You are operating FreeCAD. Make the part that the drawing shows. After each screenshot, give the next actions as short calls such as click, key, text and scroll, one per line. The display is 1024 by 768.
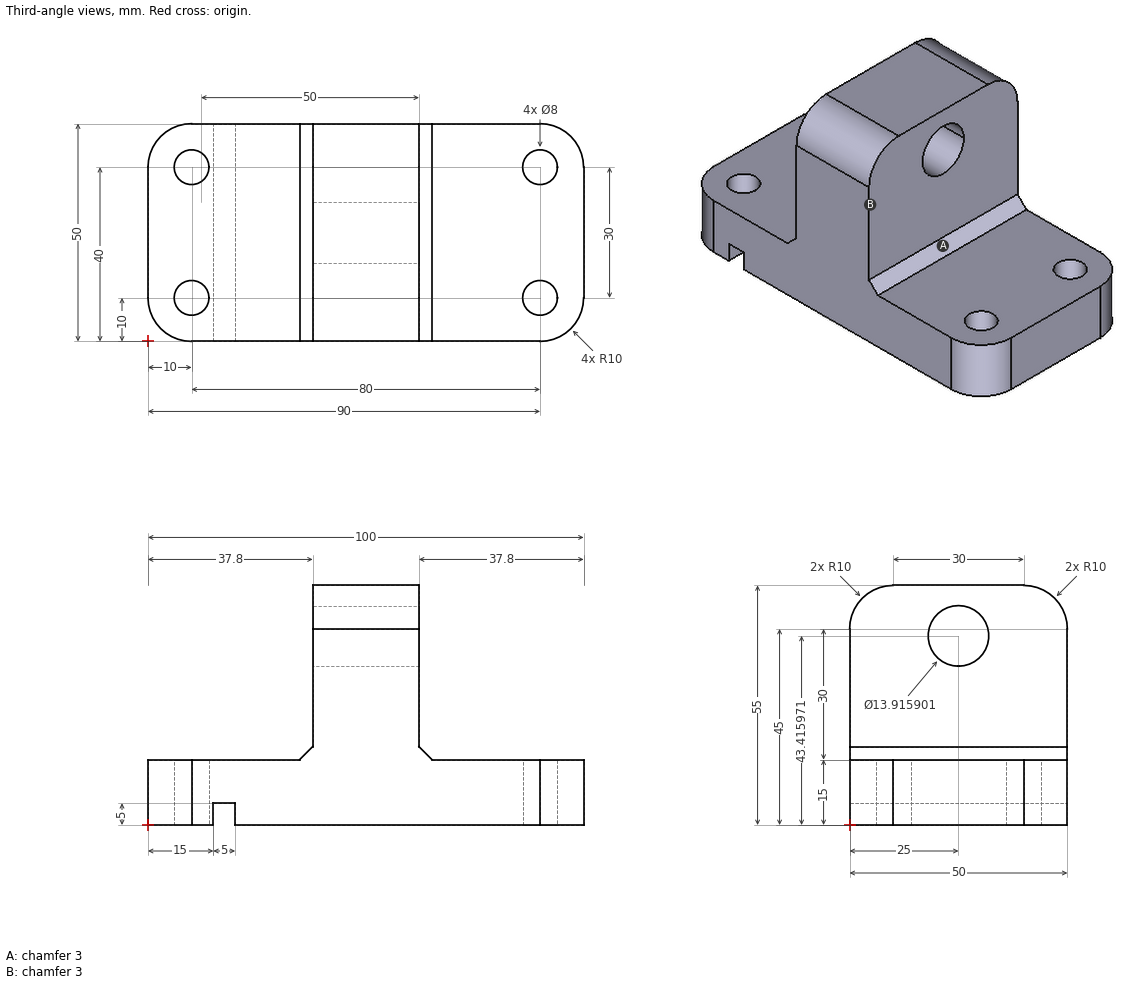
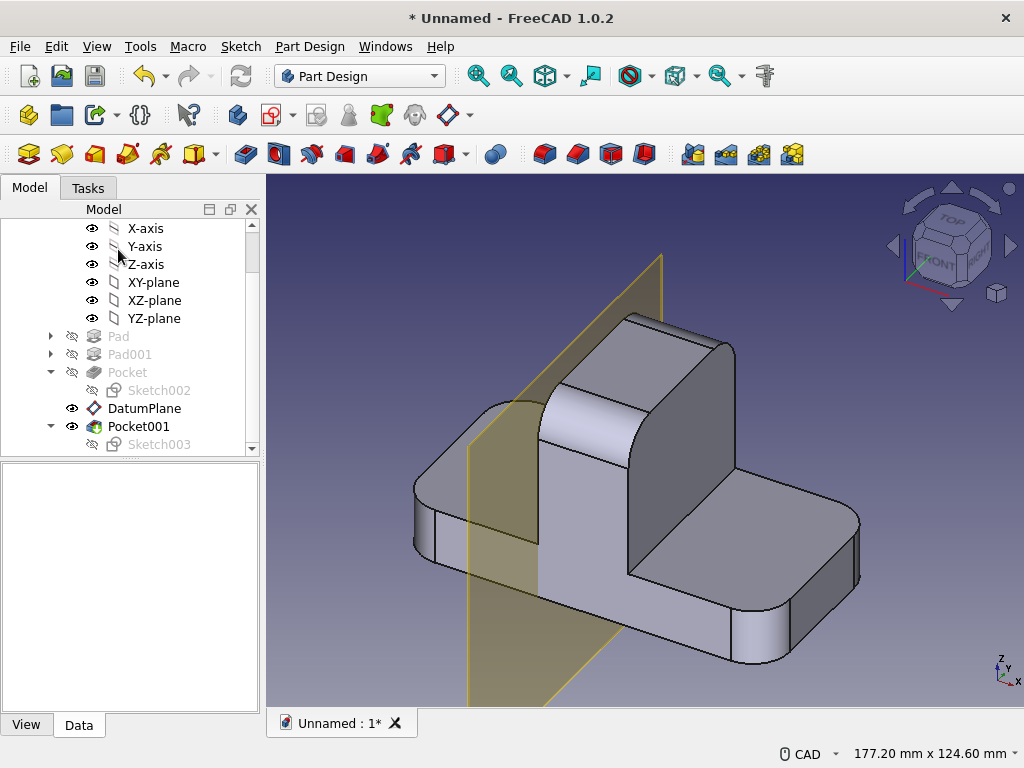
click(117, 408)
key(space)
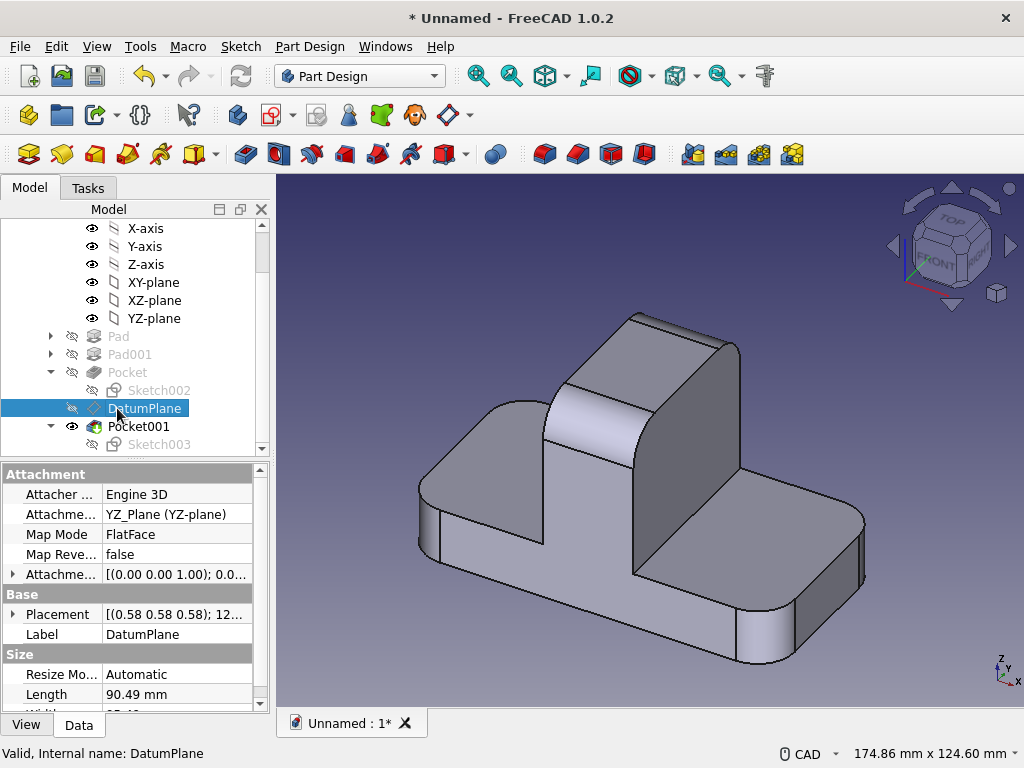
click(316, 667)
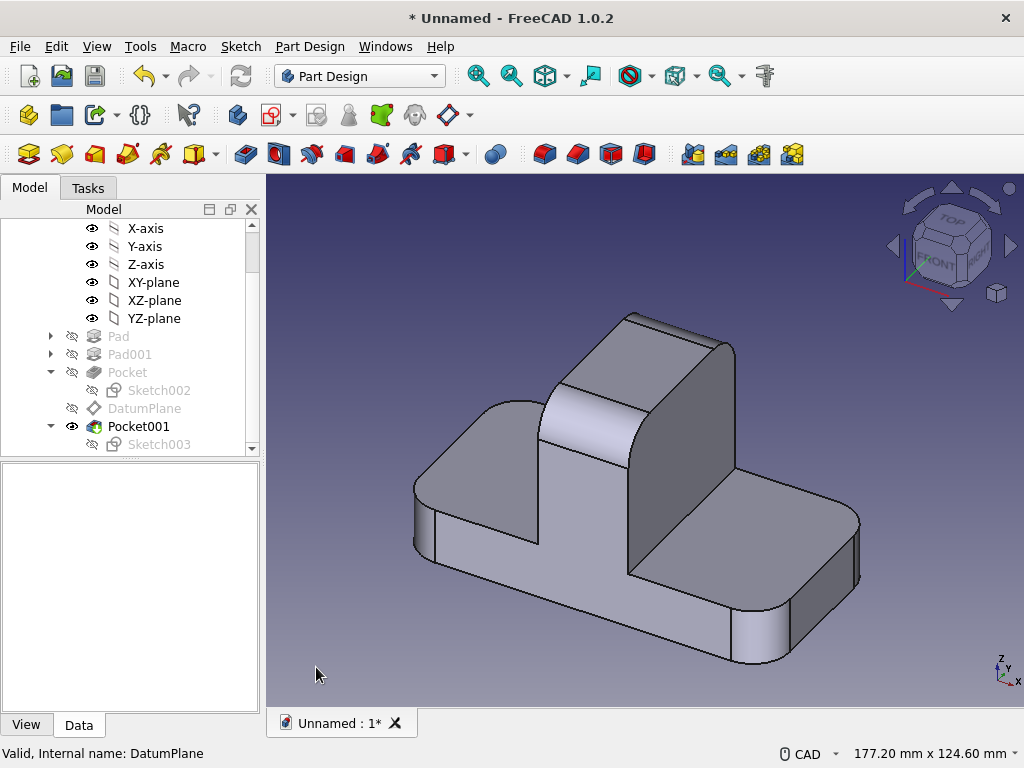
click(270, 116)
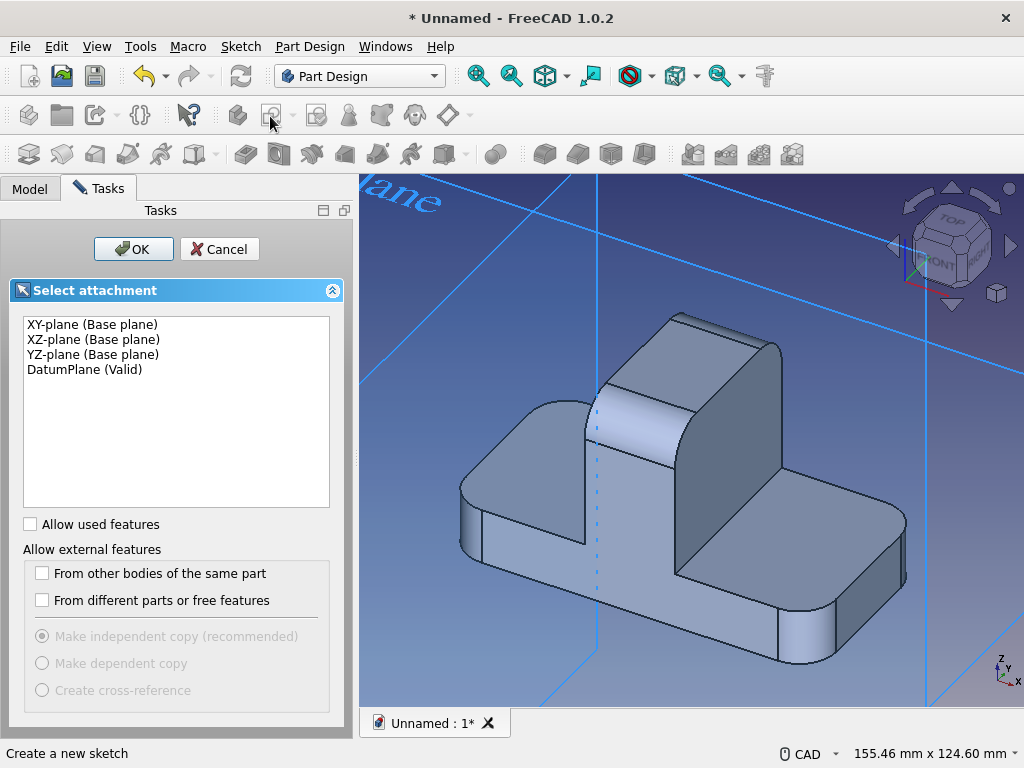
click(84, 340)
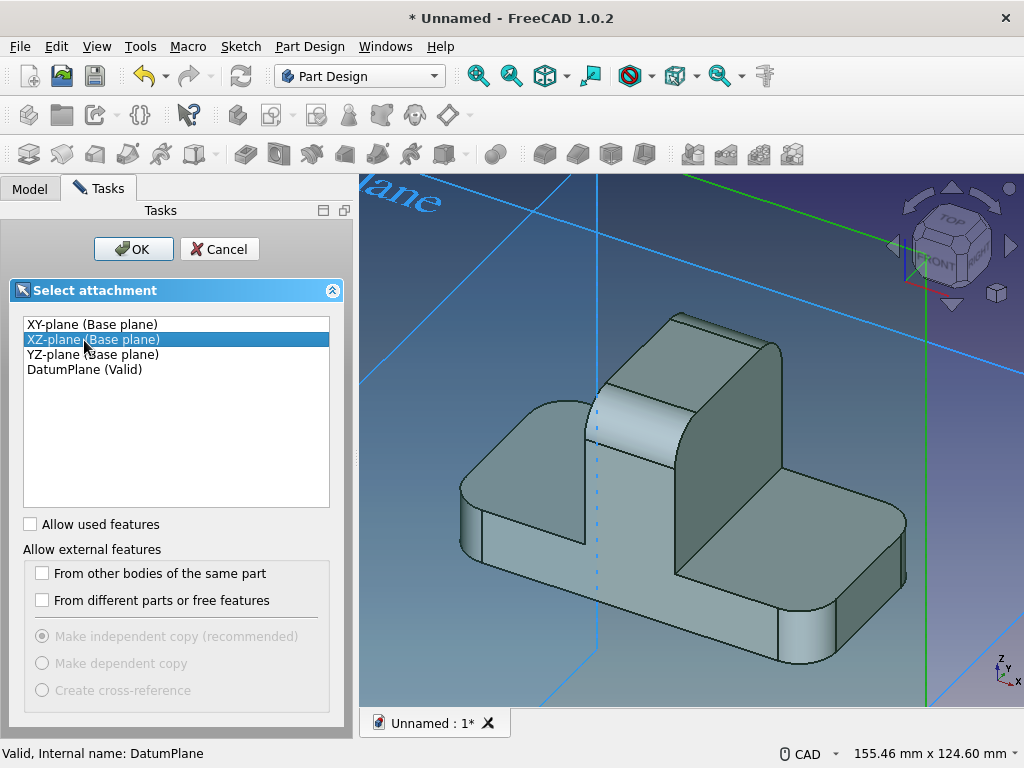
click(134, 249)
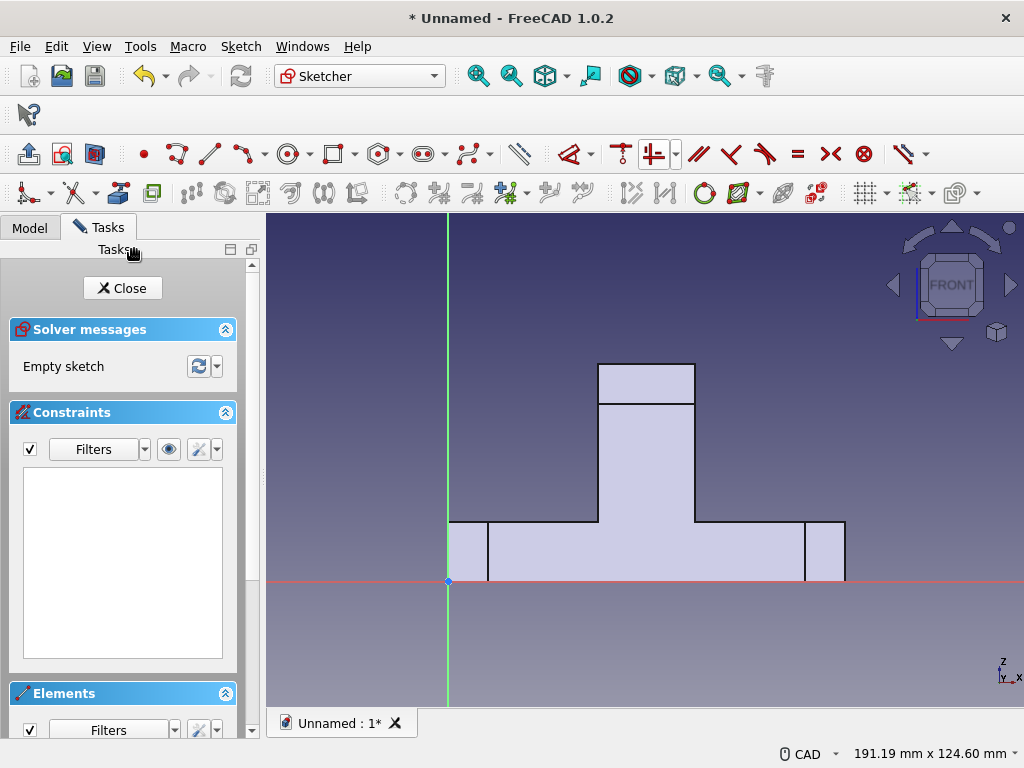
scroll(514, 579, up, 14)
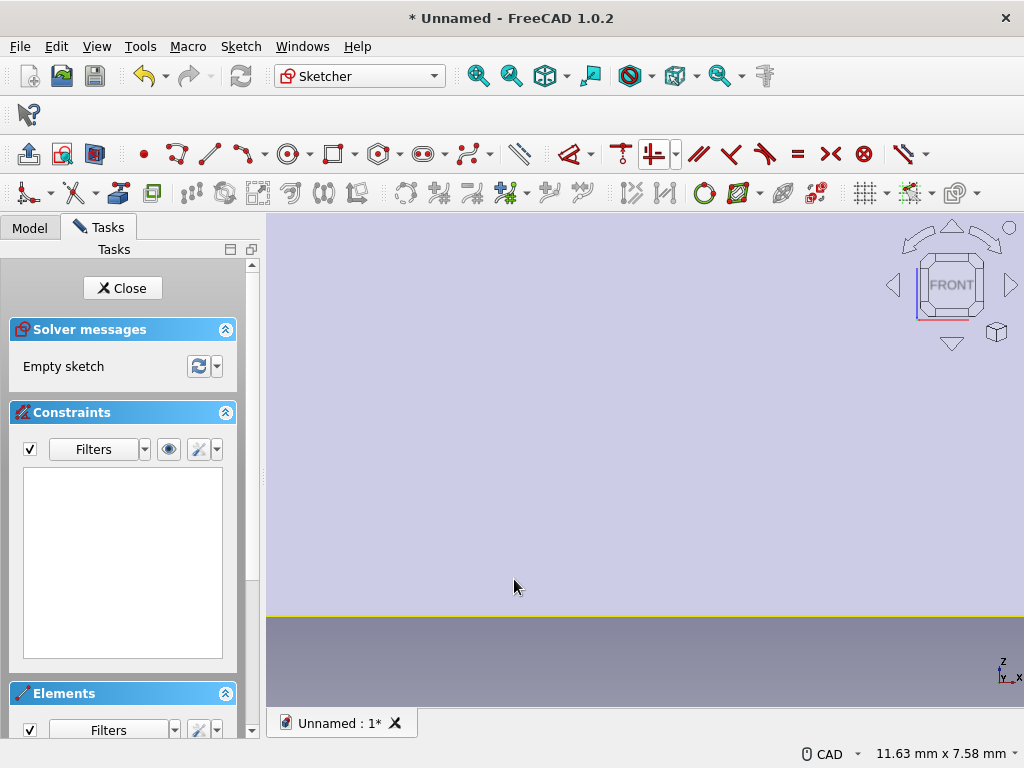
click(332, 154)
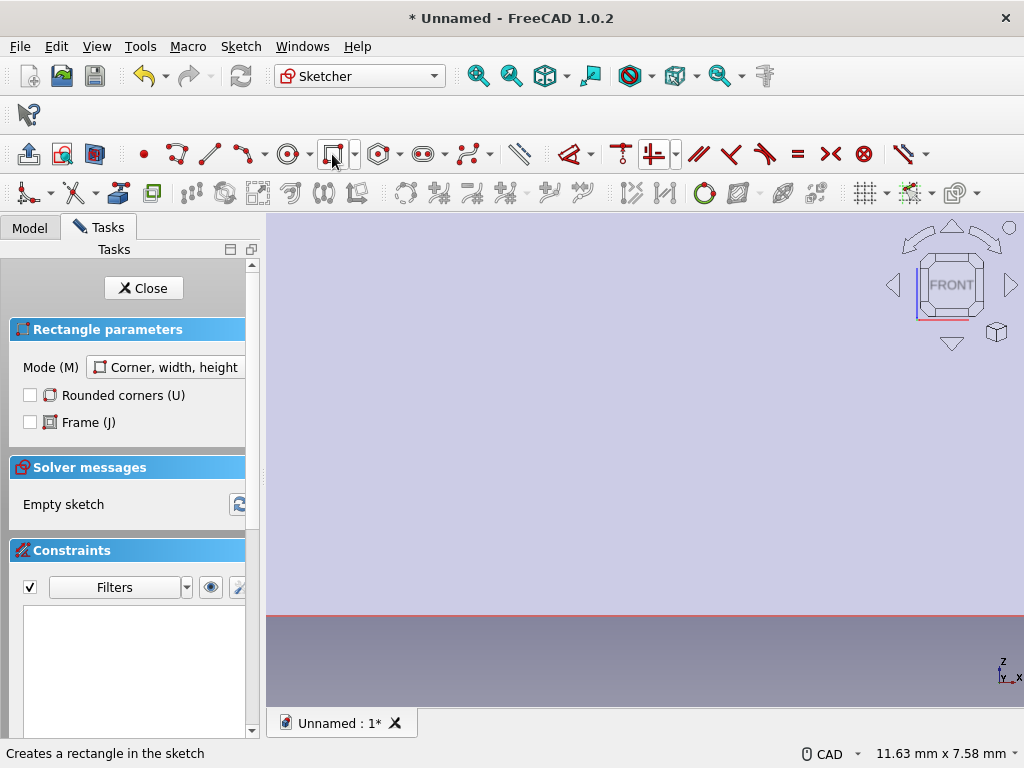
click(409, 290)
click(735, 616)
key(Escape)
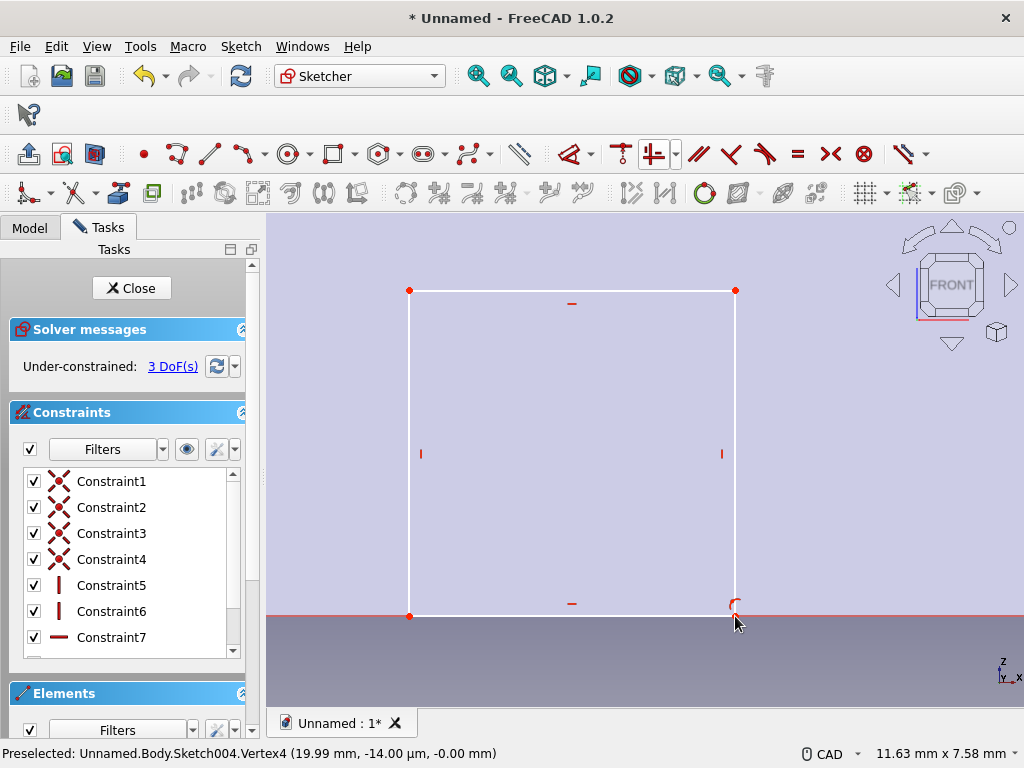
click(568, 154)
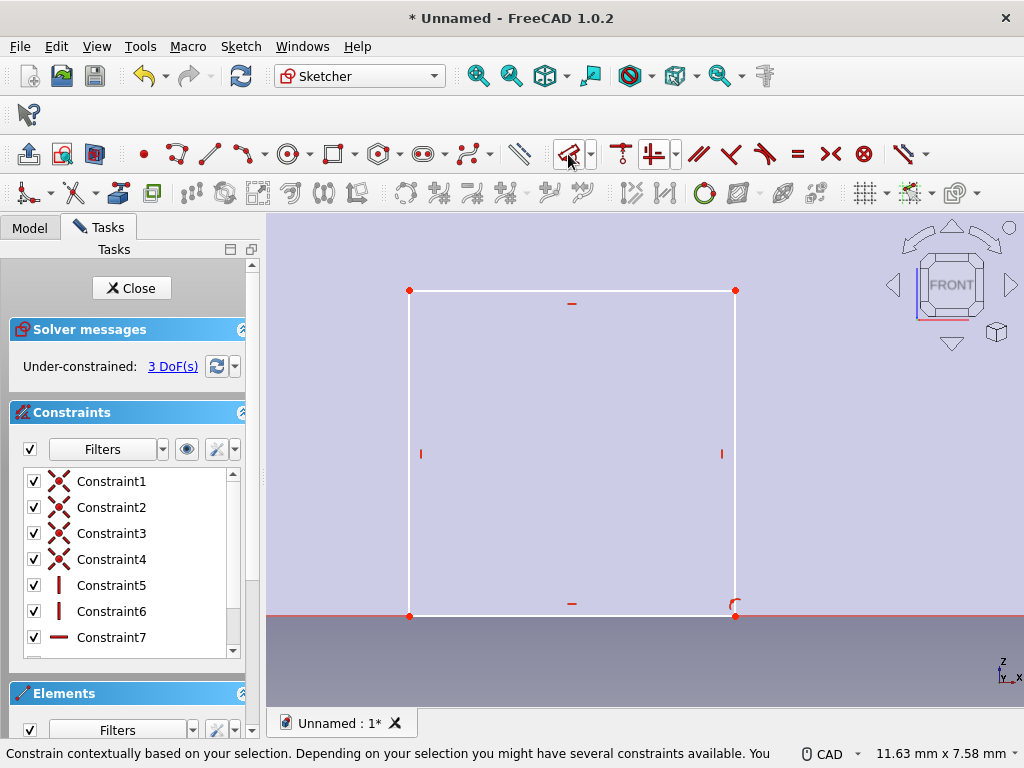
click(409, 389)
click(375, 454)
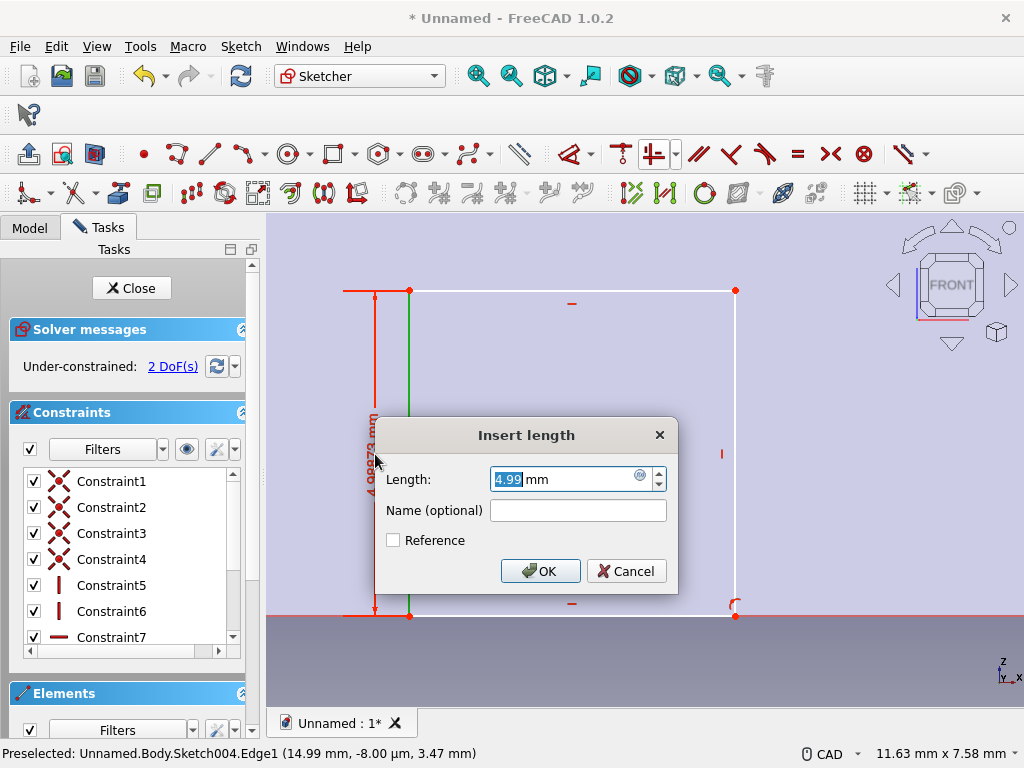
text(5)
key(Return)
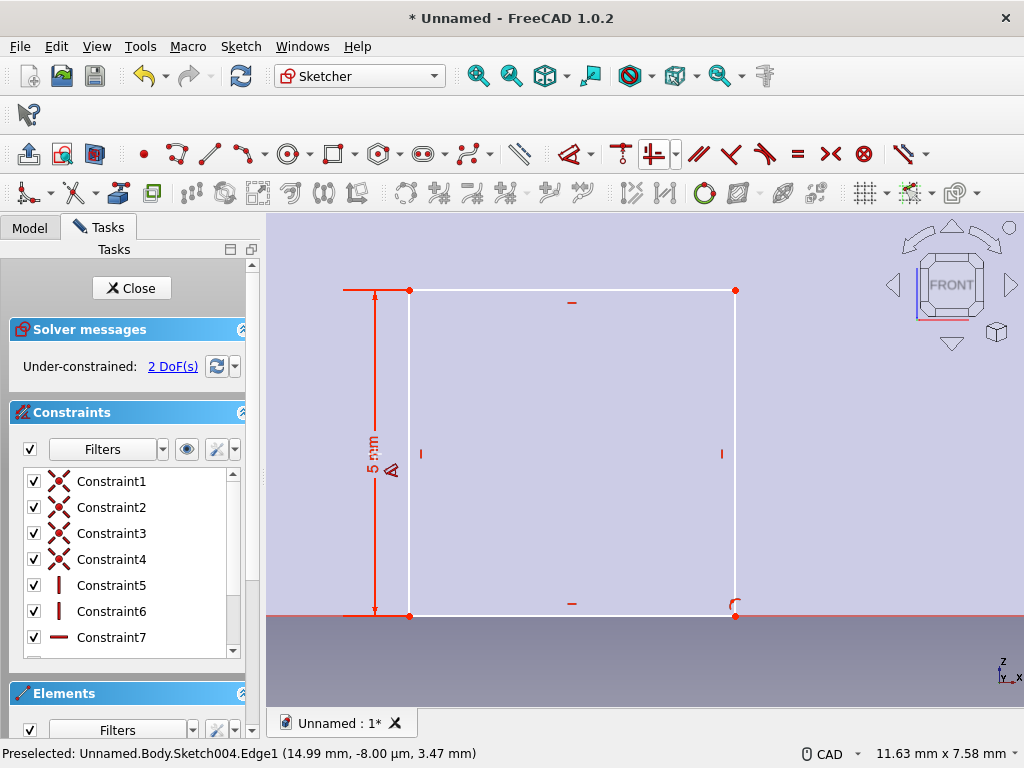
click(507, 616)
click(572, 650)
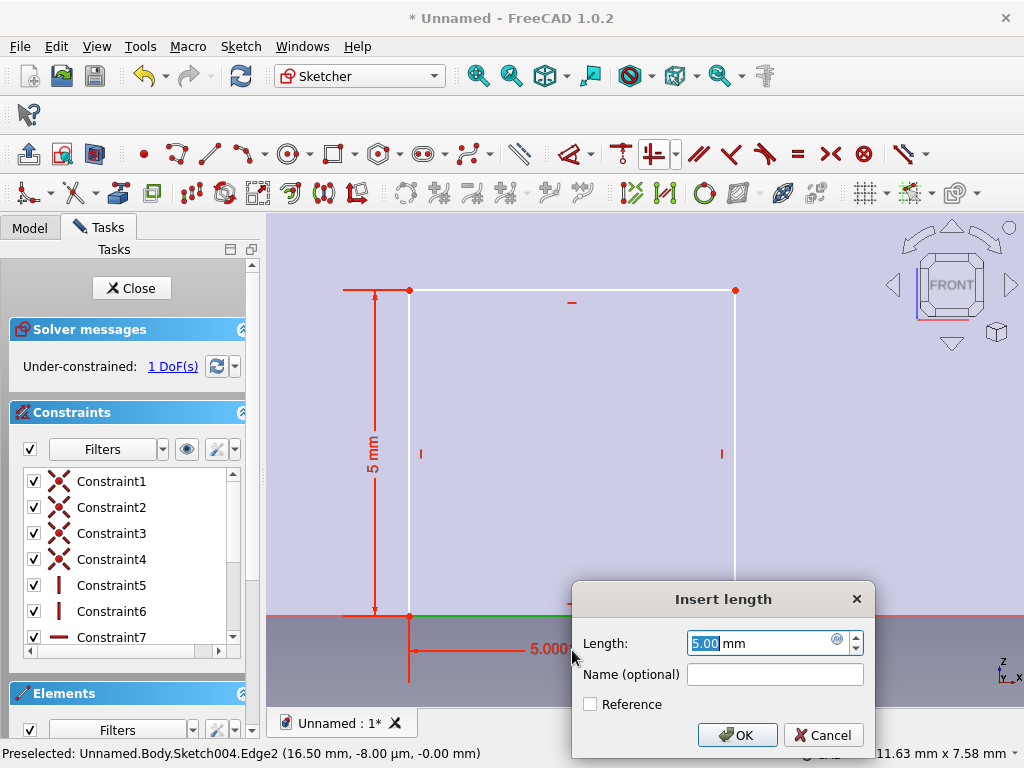
text(5)
key(Return)